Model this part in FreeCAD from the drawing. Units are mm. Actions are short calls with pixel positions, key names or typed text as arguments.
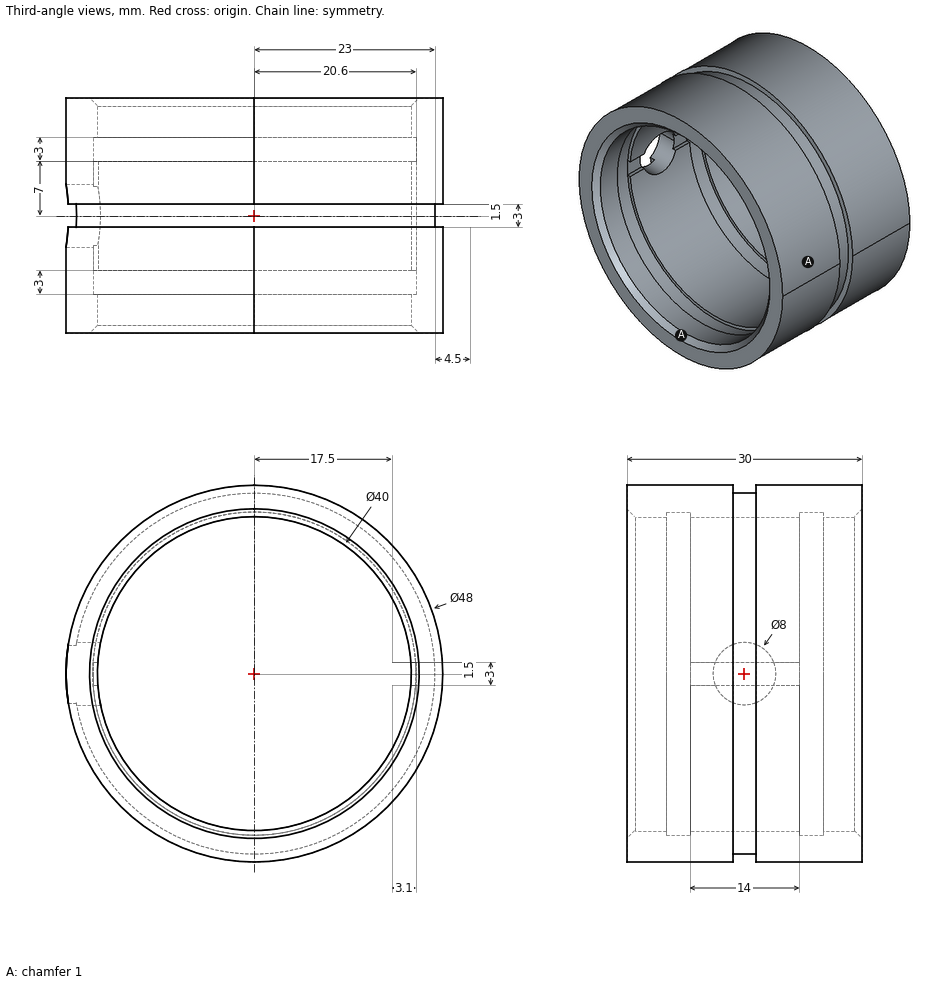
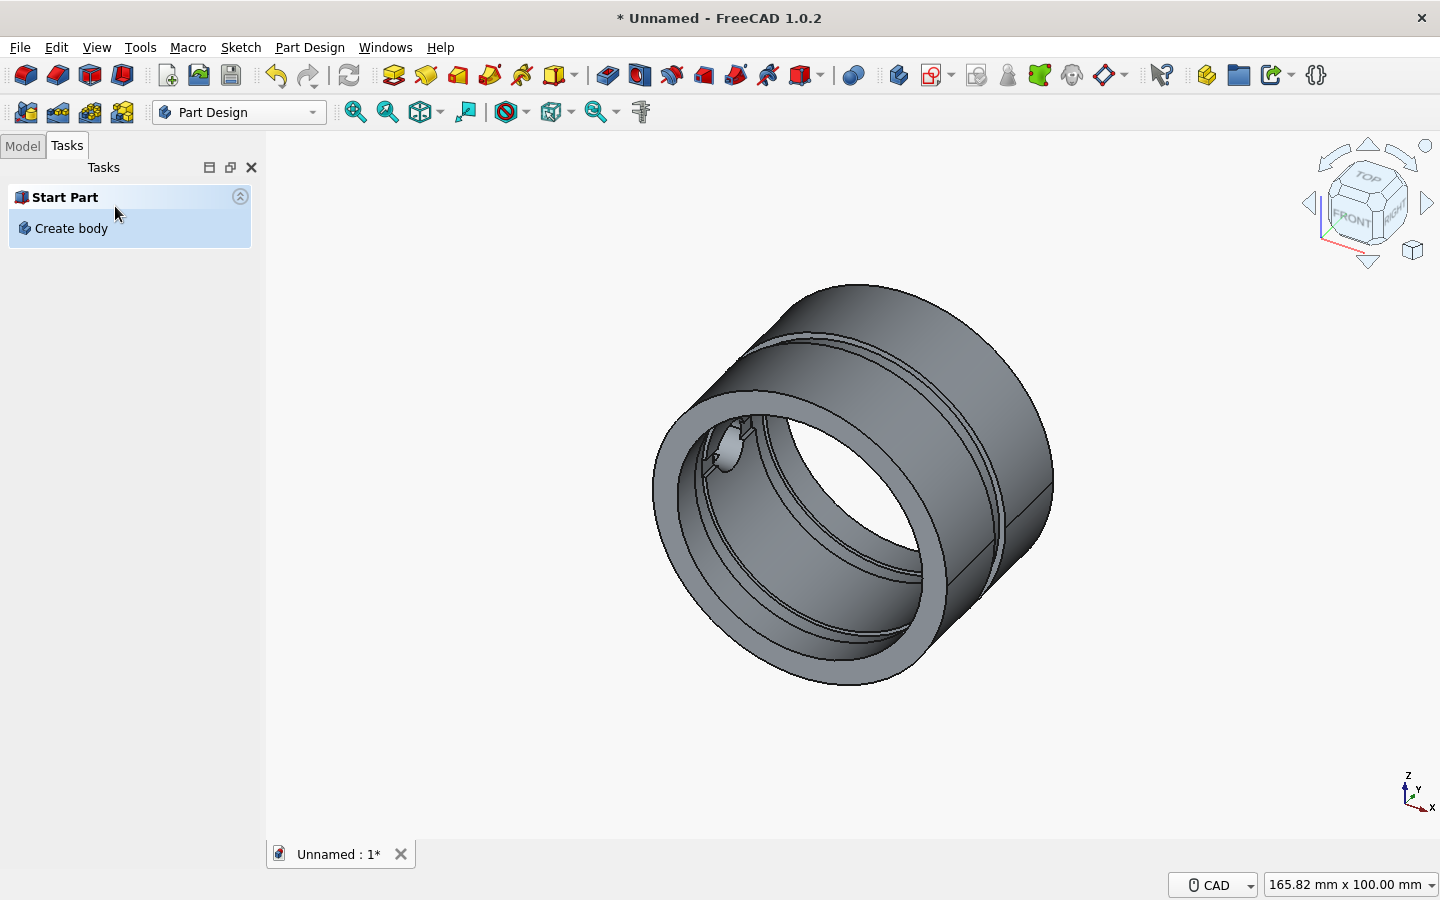
click(677, 496)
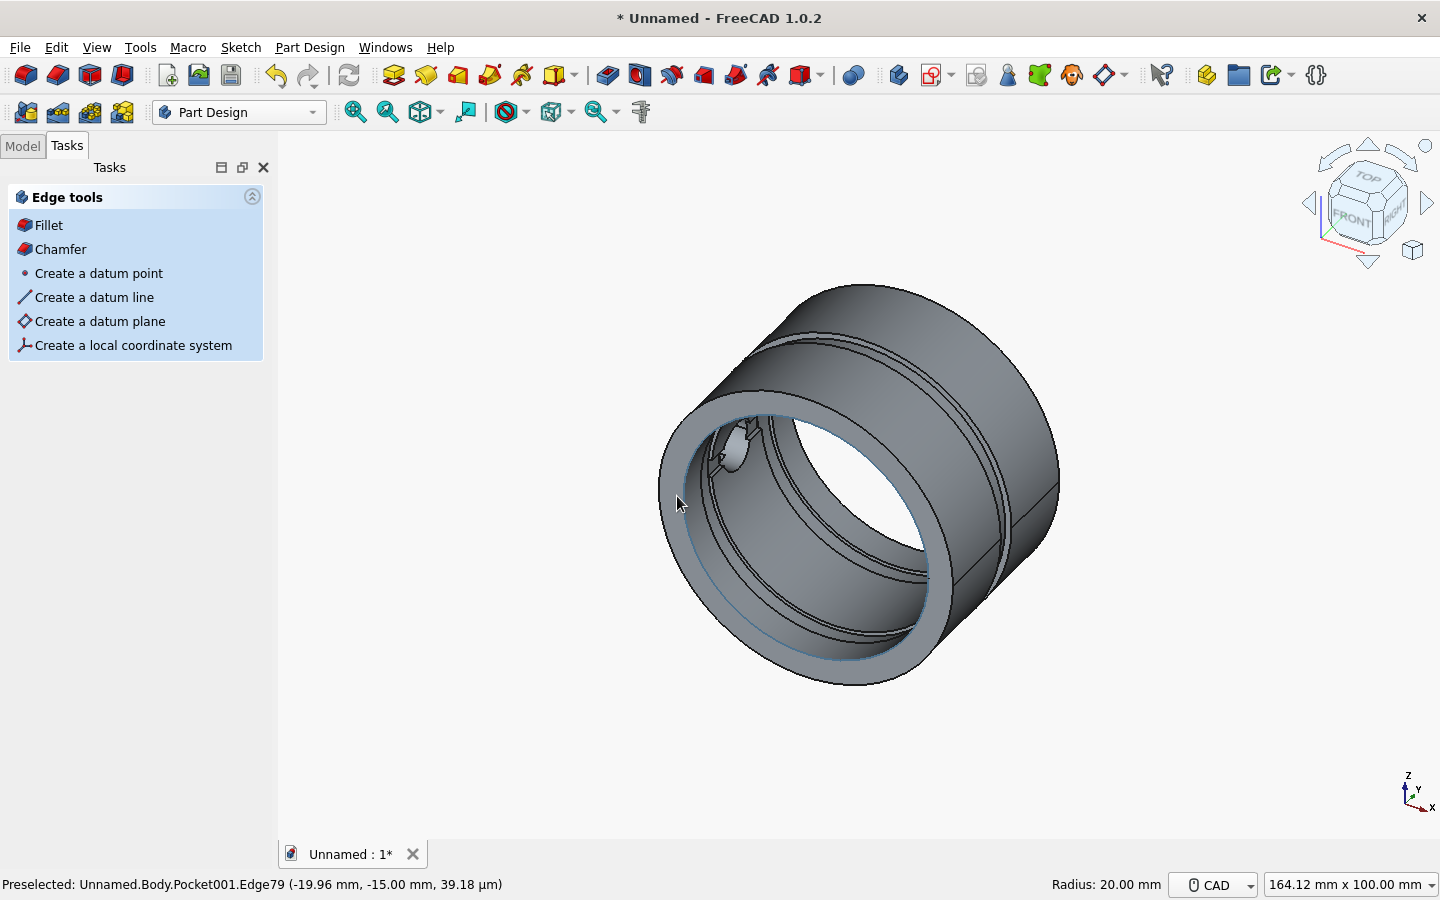
key(0)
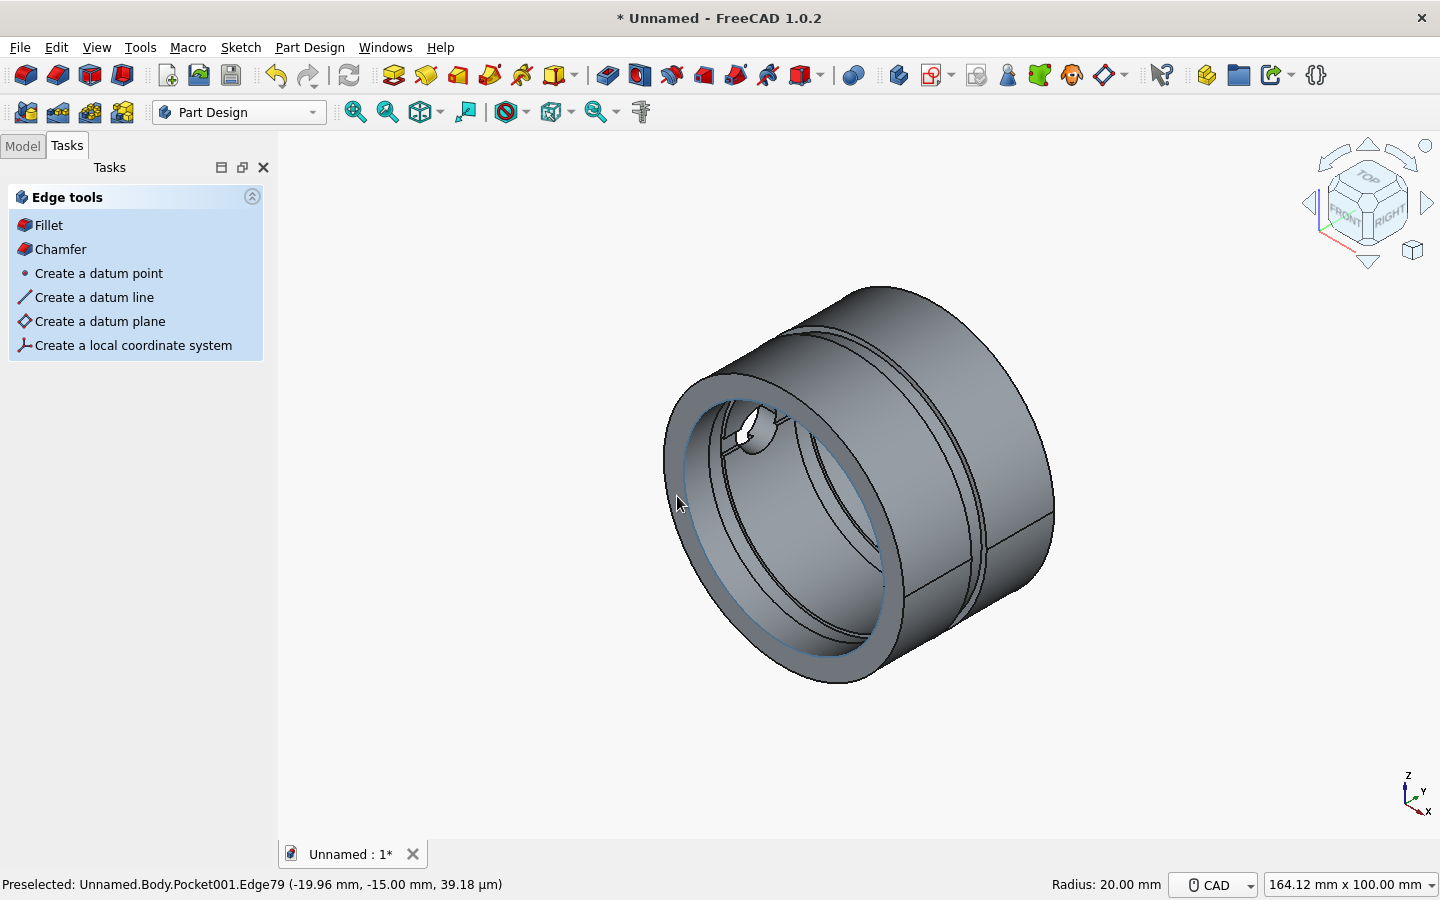
key(2)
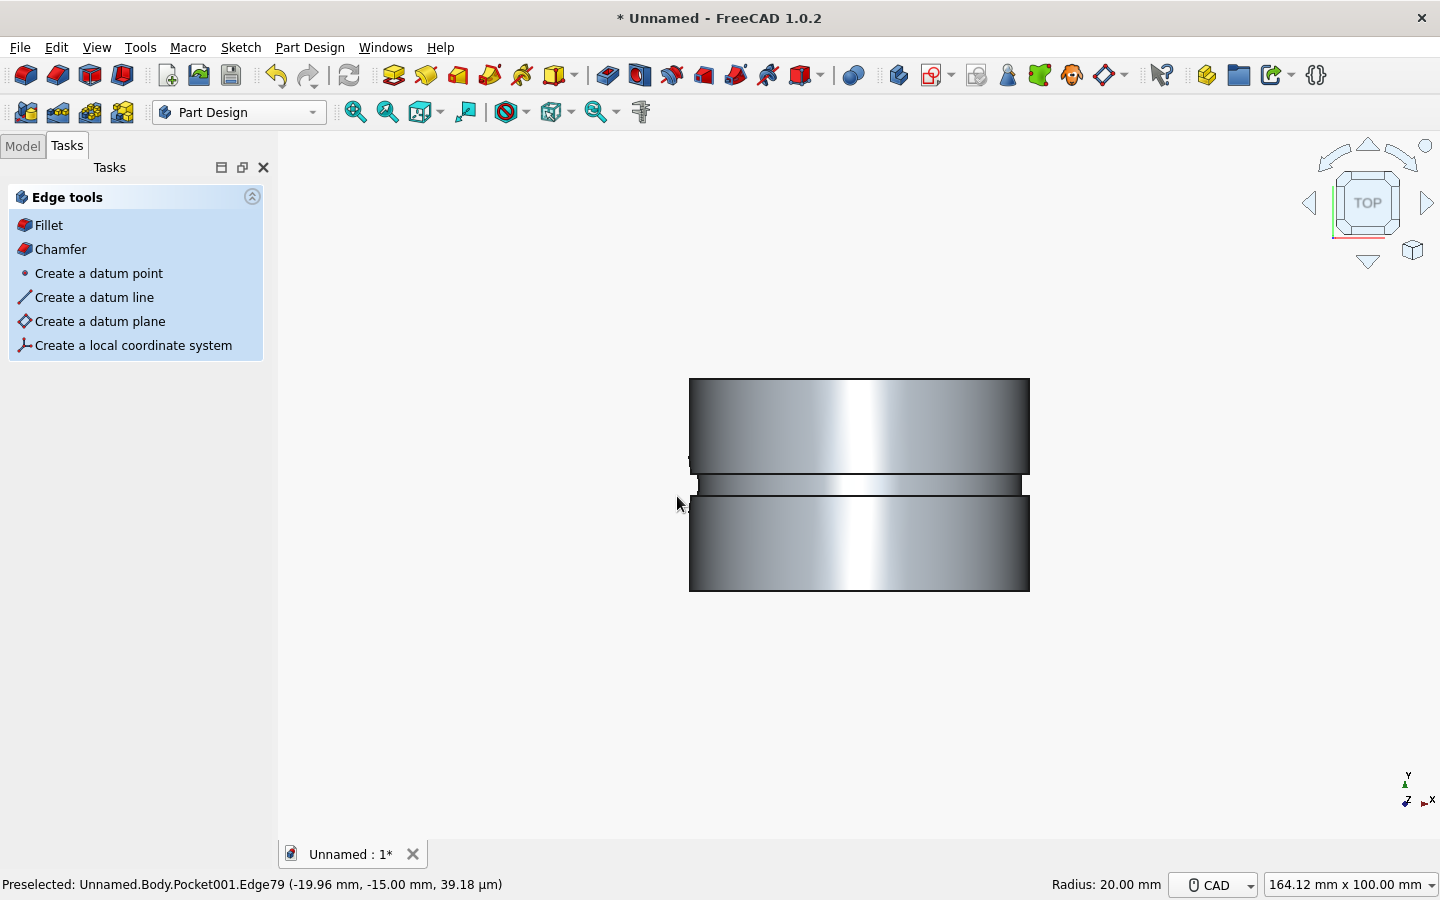
key(v)
key(f)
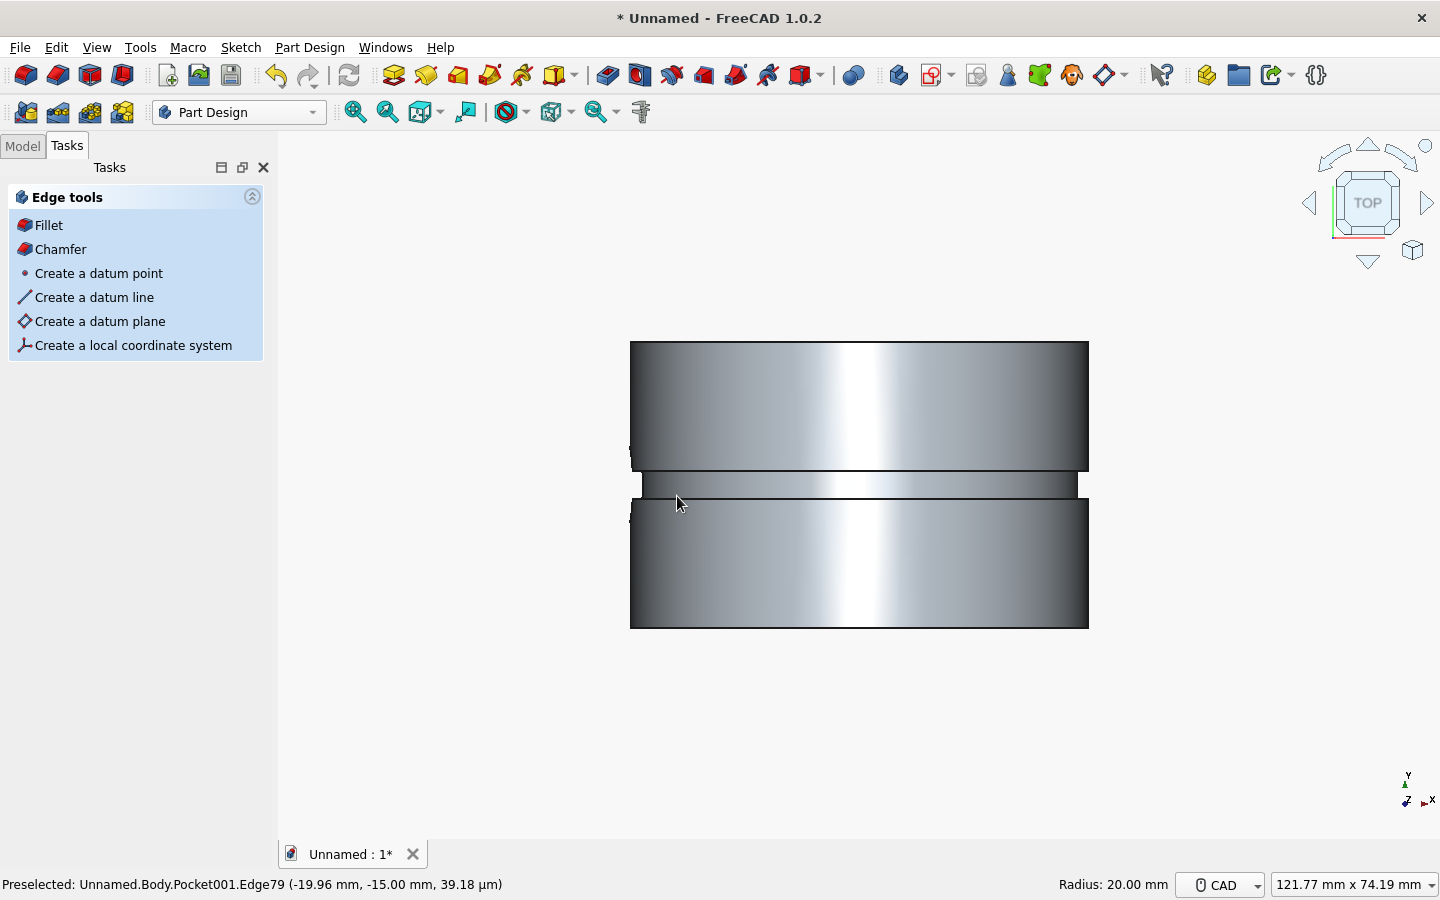
key(1)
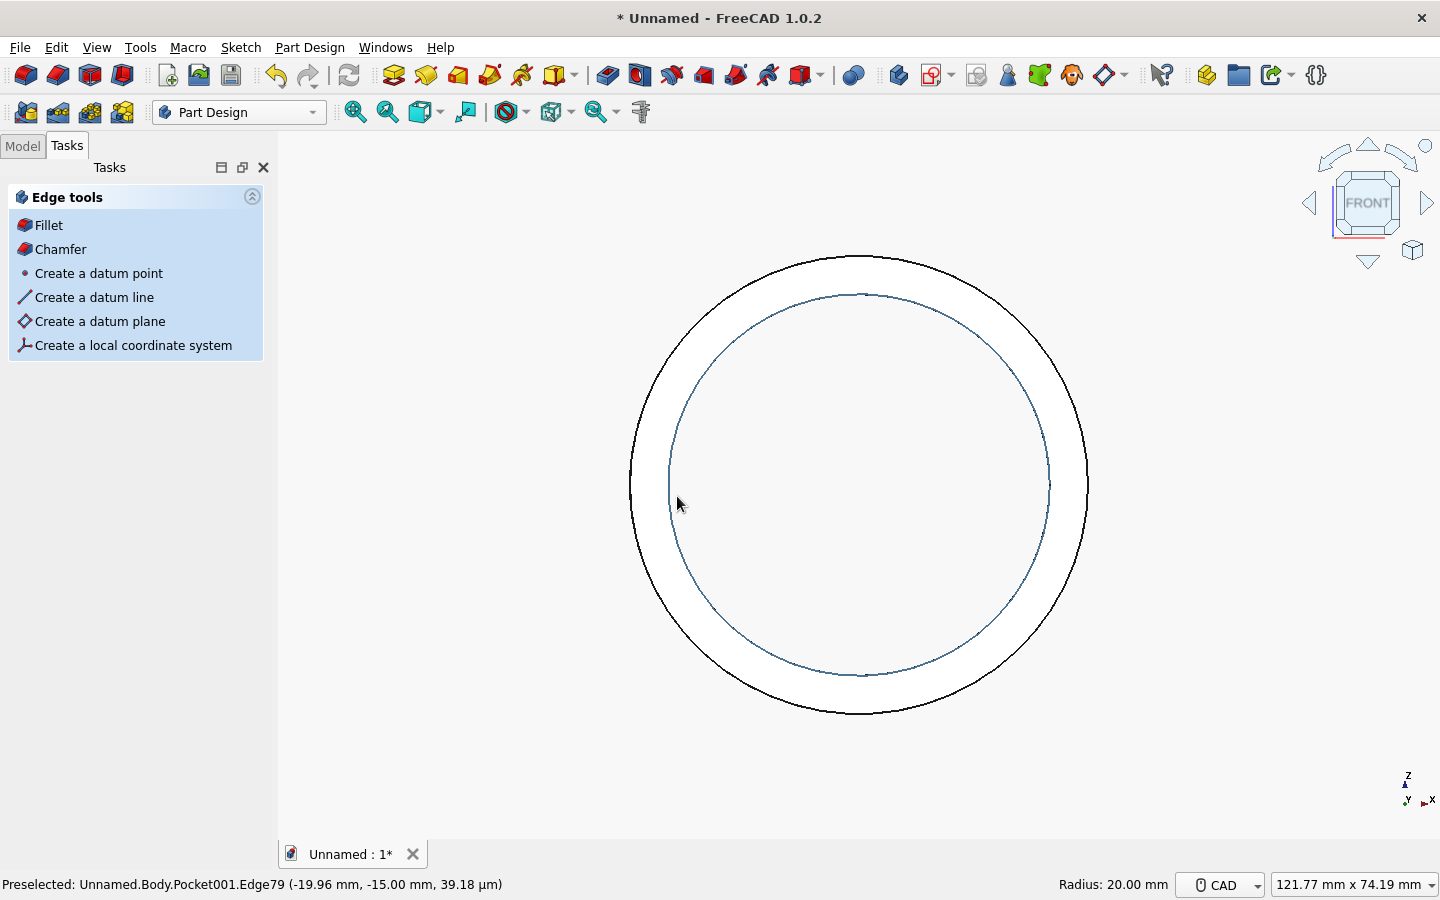
key(3)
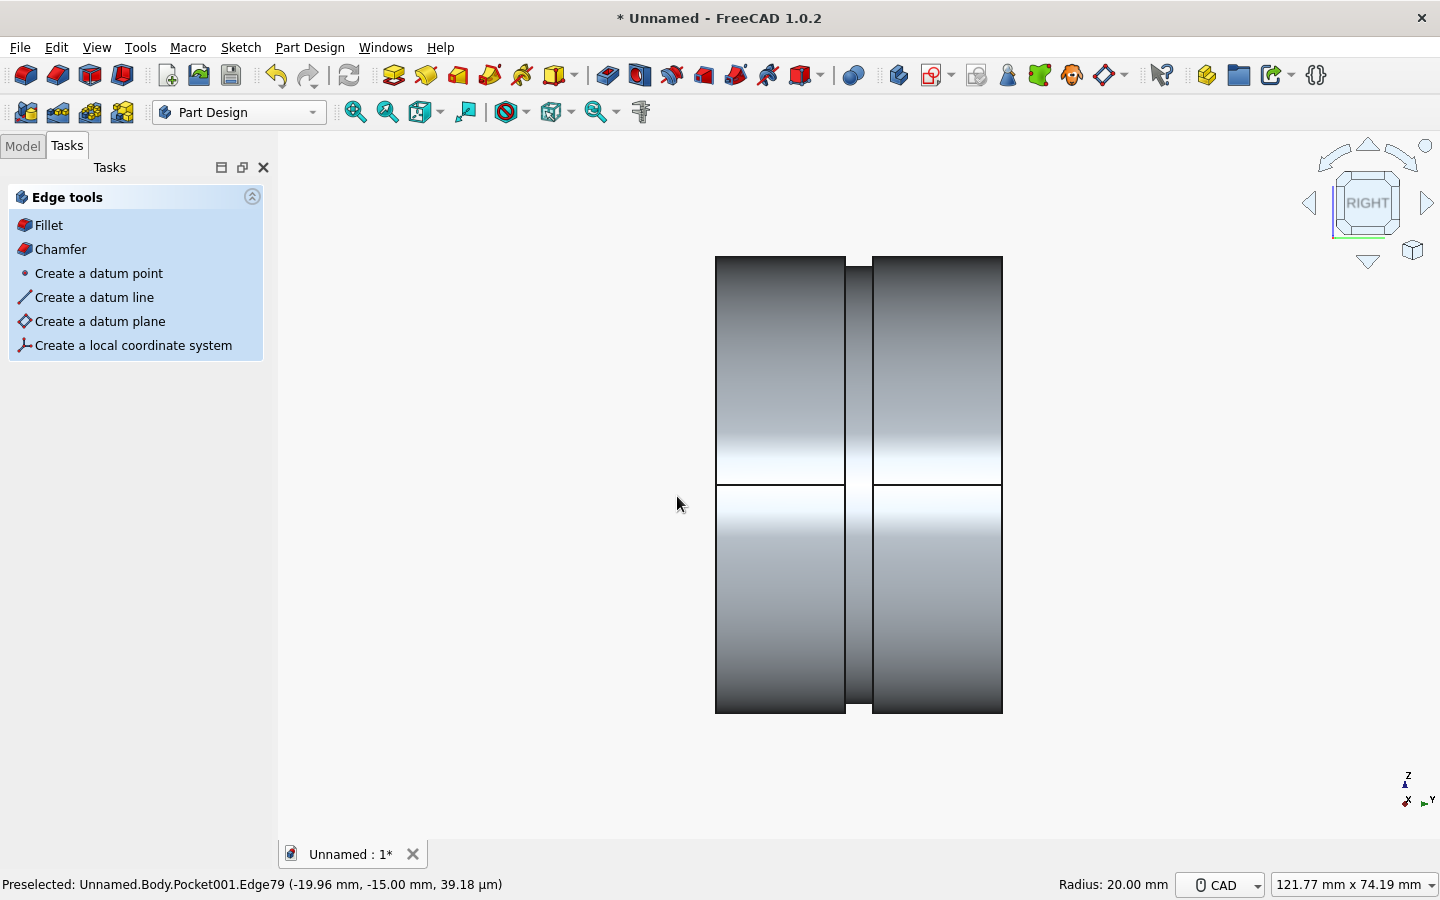
key(5)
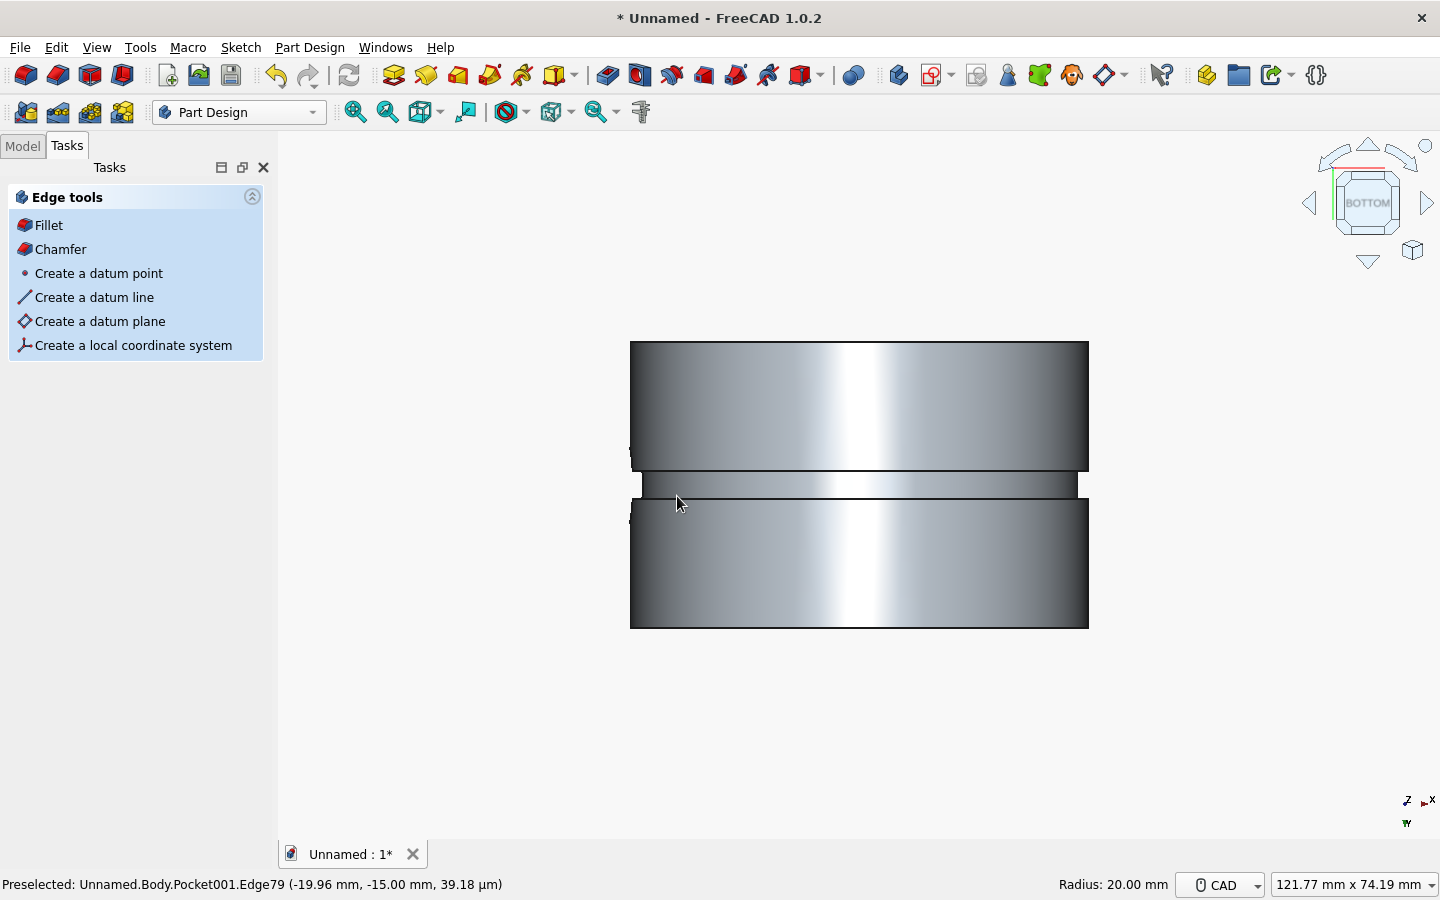
click(356, 112)